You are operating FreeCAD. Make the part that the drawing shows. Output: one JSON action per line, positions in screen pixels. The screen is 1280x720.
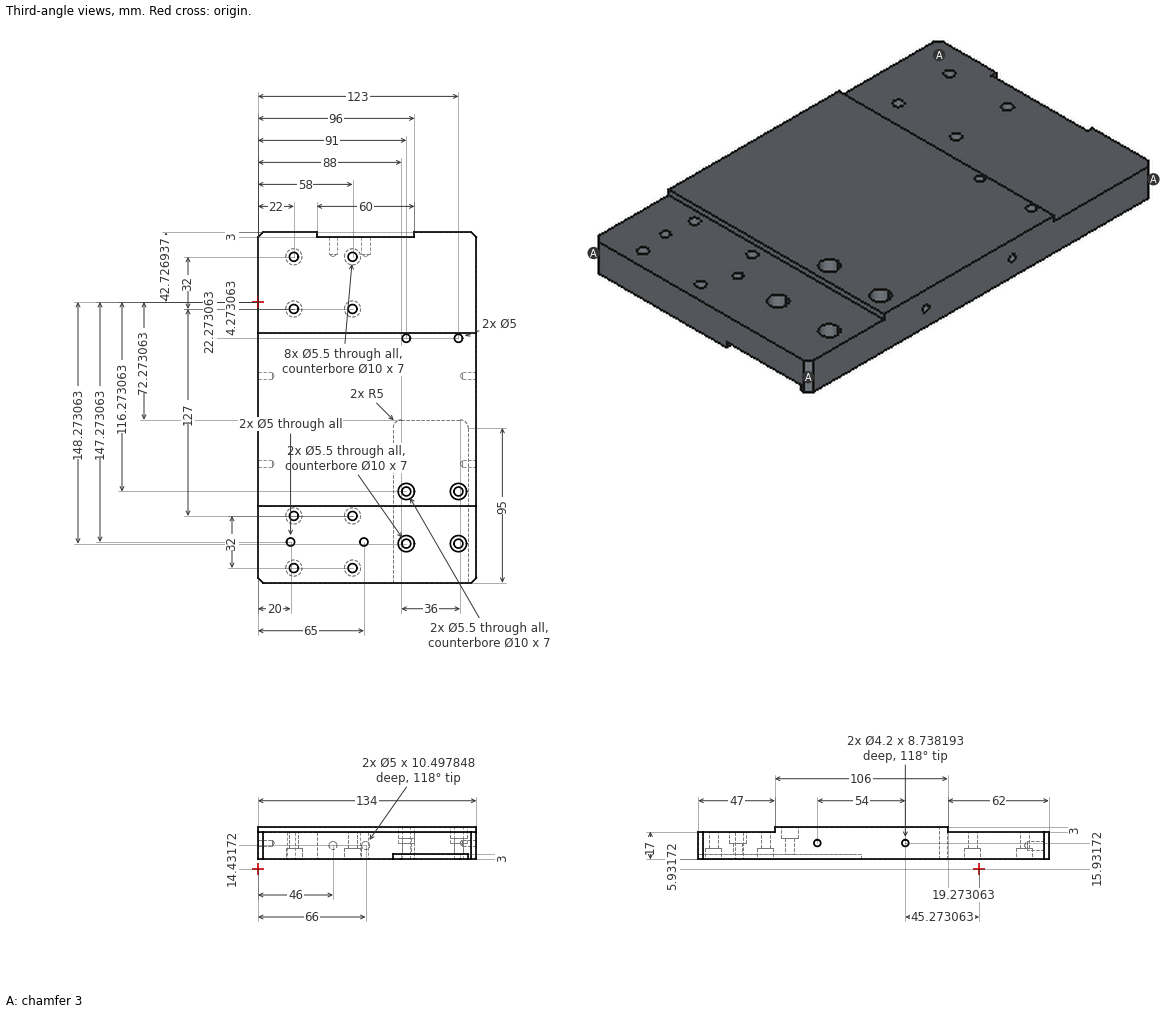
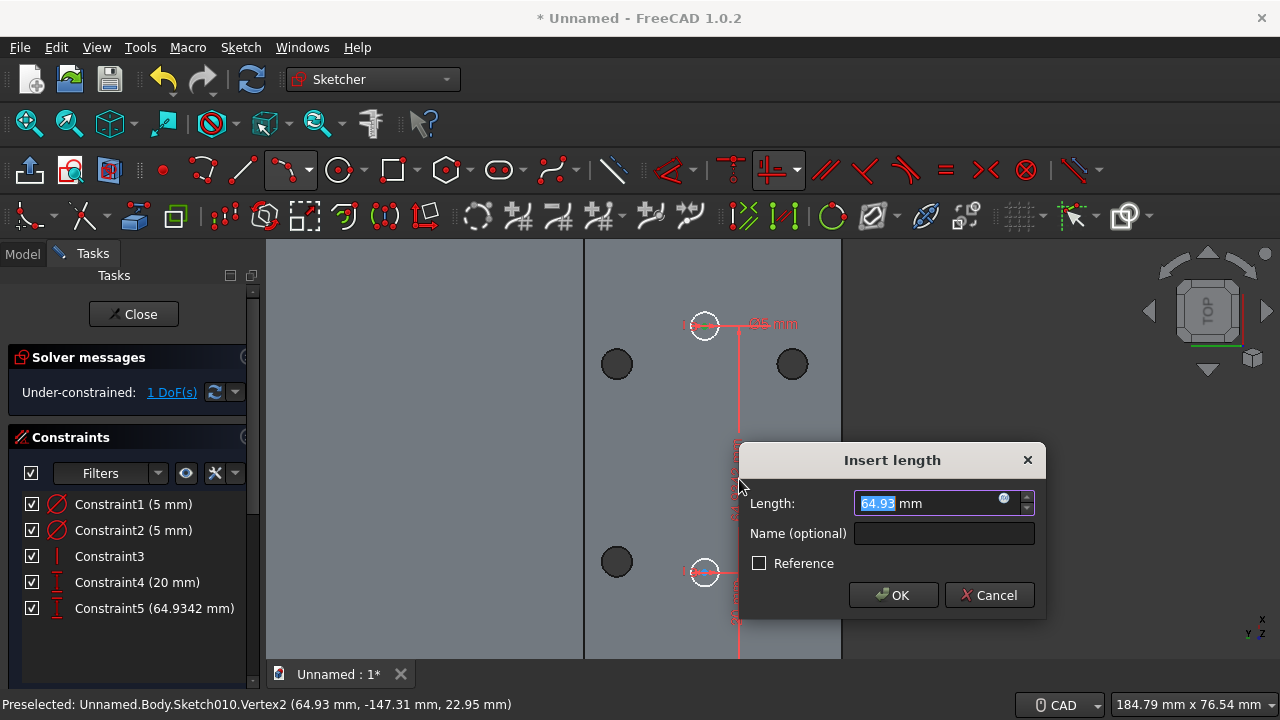
{"action": "type", "text": "65"}
{"action": "key", "text": "Return"}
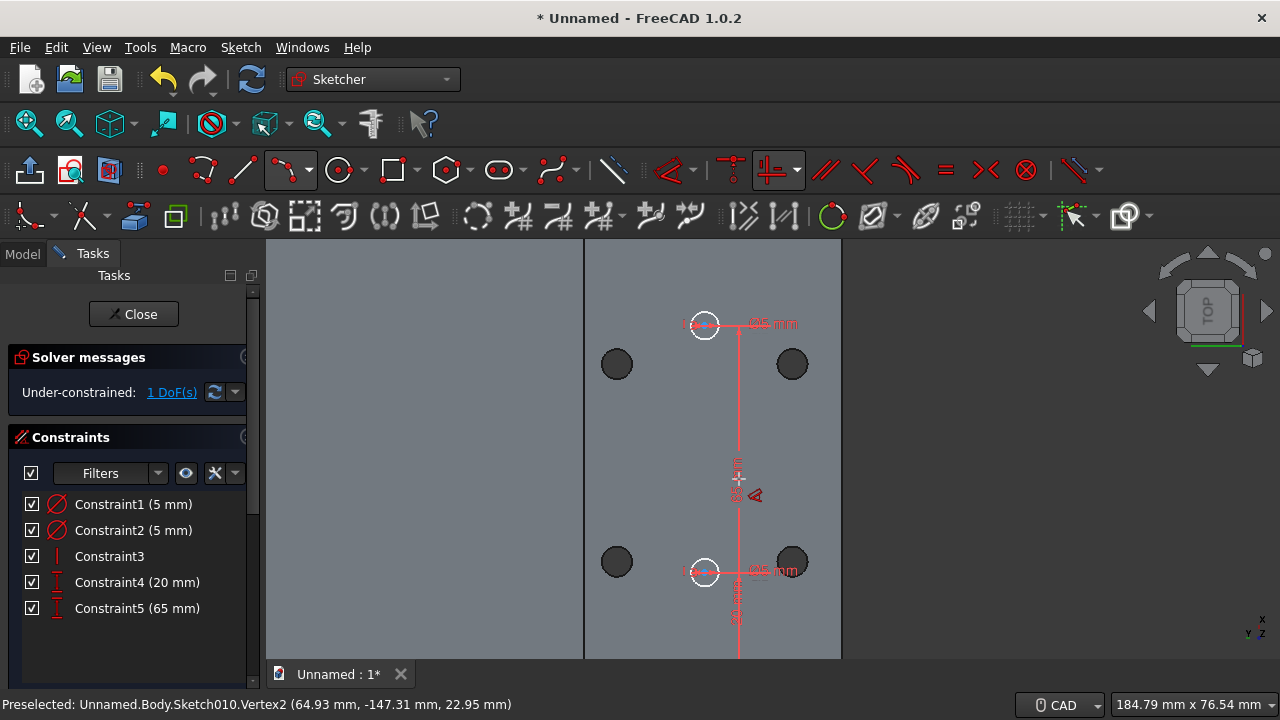
{"action": "left_click", "coordinate": [705, 573]}
{"action": "left_click", "coordinate": [499, 539]}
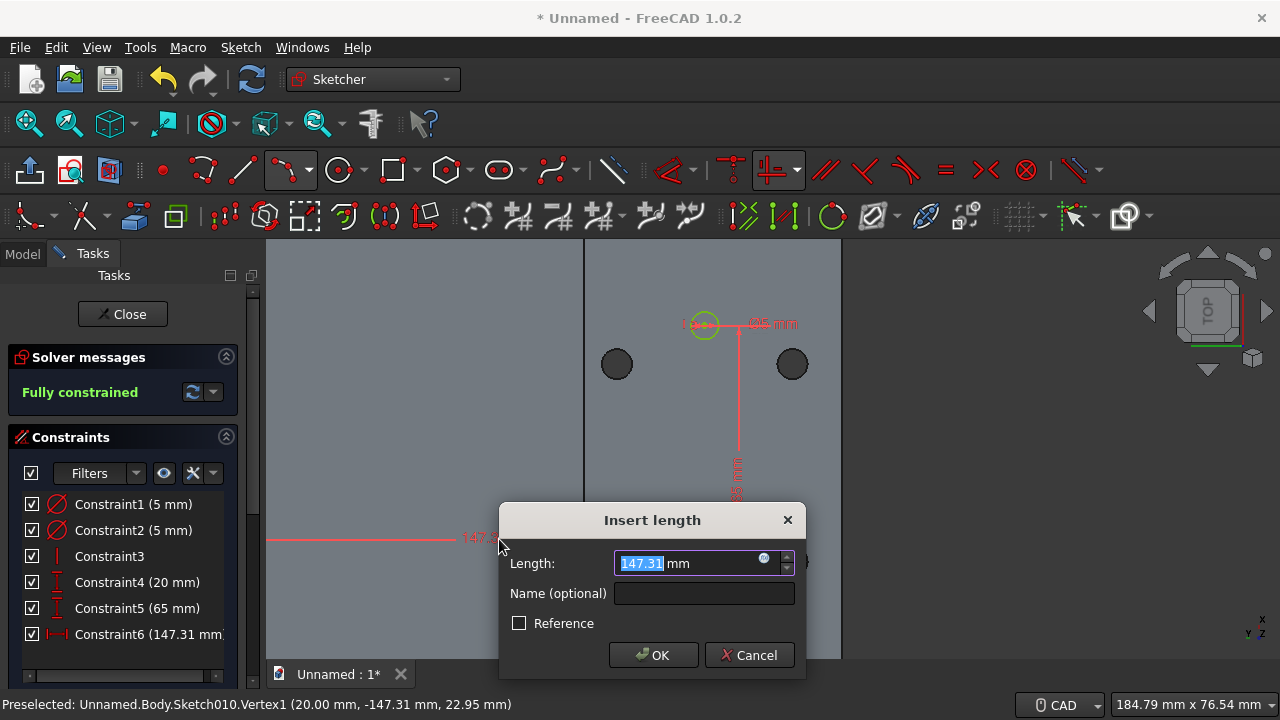
{"action": "type", "text": "147.273063"}
{"action": "key", "text": "Return"}
{"action": "key", "text": "Escape"}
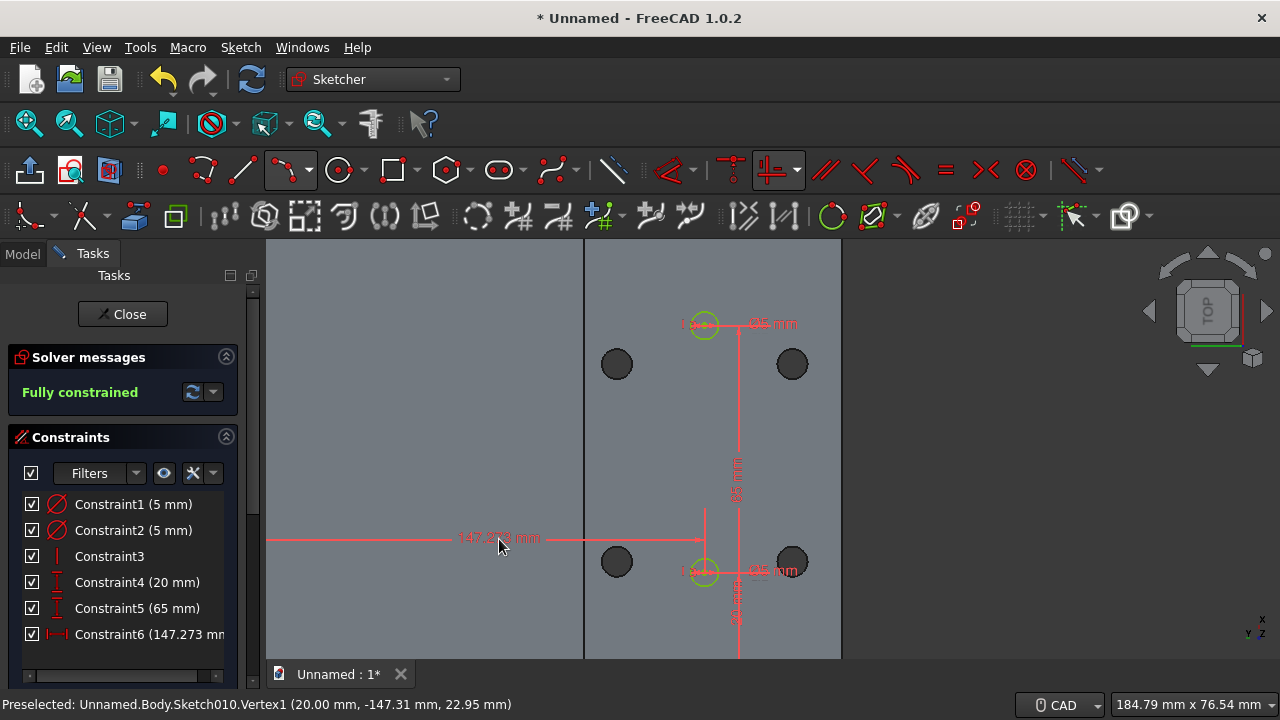
{"action": "left_click", "coordinate": [123, 314]}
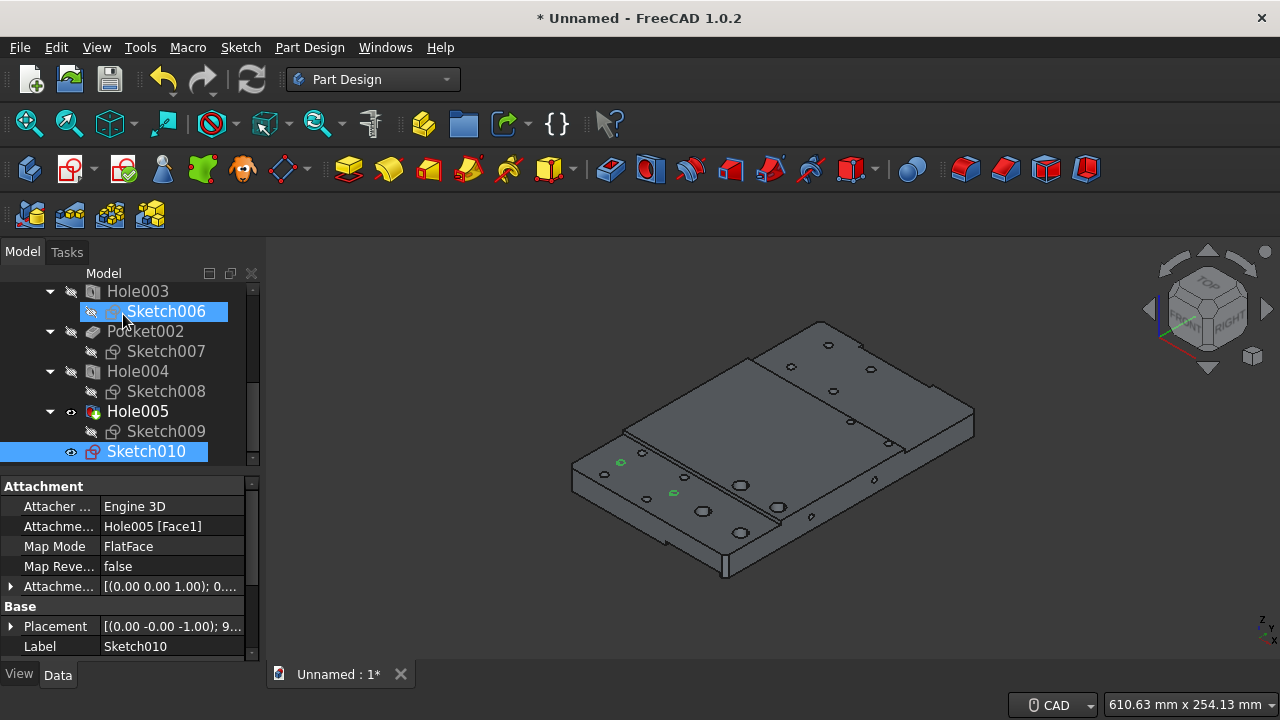
{"action": "left_click", "coordinate": [652, 170]}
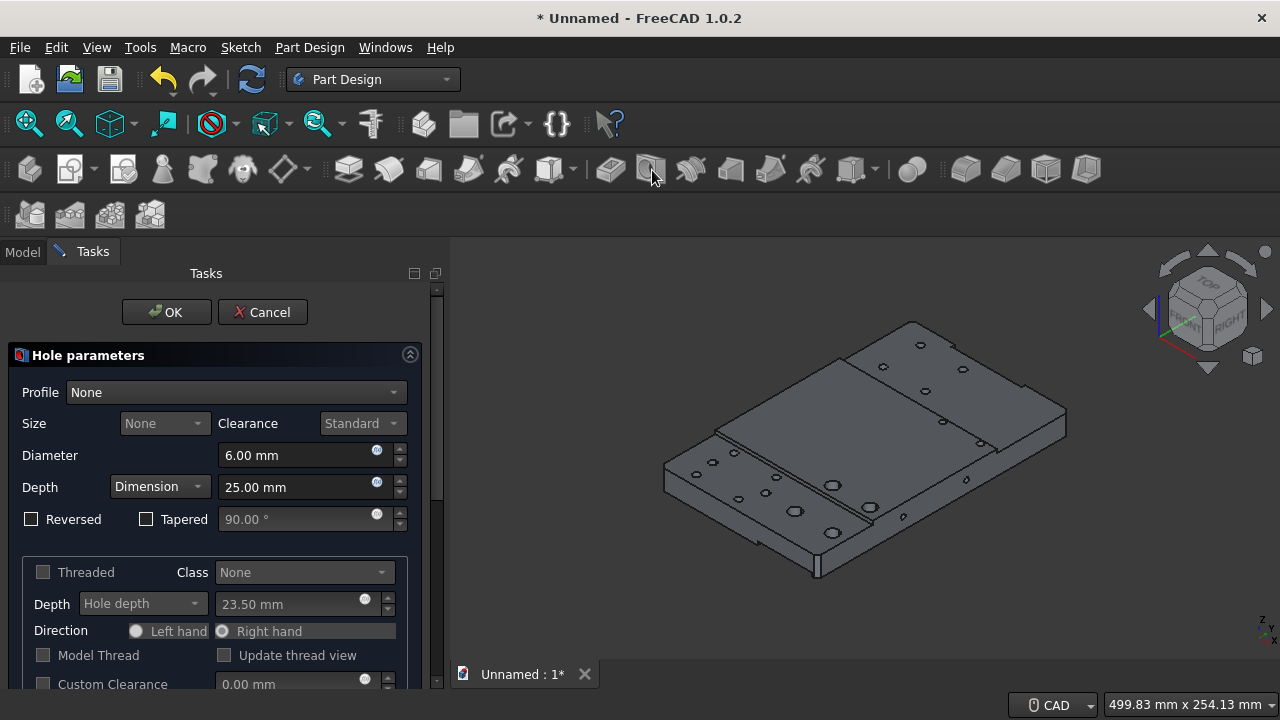
{"action": "triple_click", "coordinate": [305, 455]}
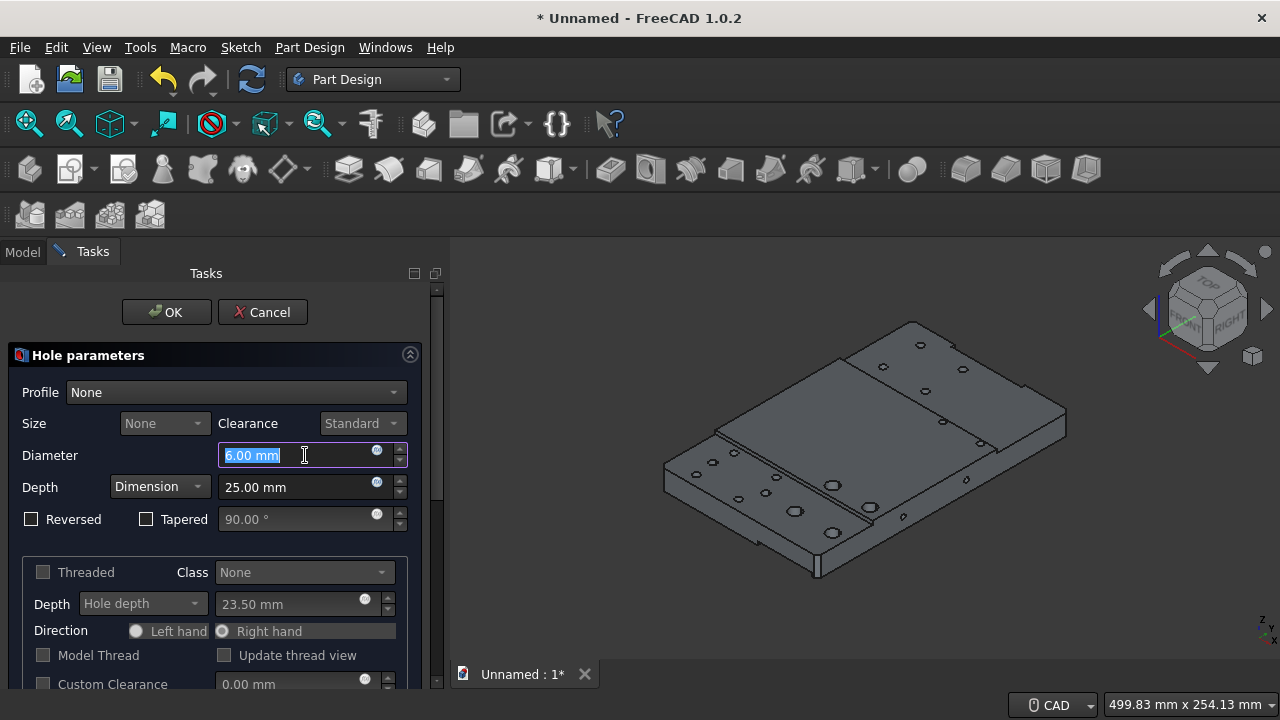
{"action": "type", "text": "5"}
{"action": "key", "text": "Tab"}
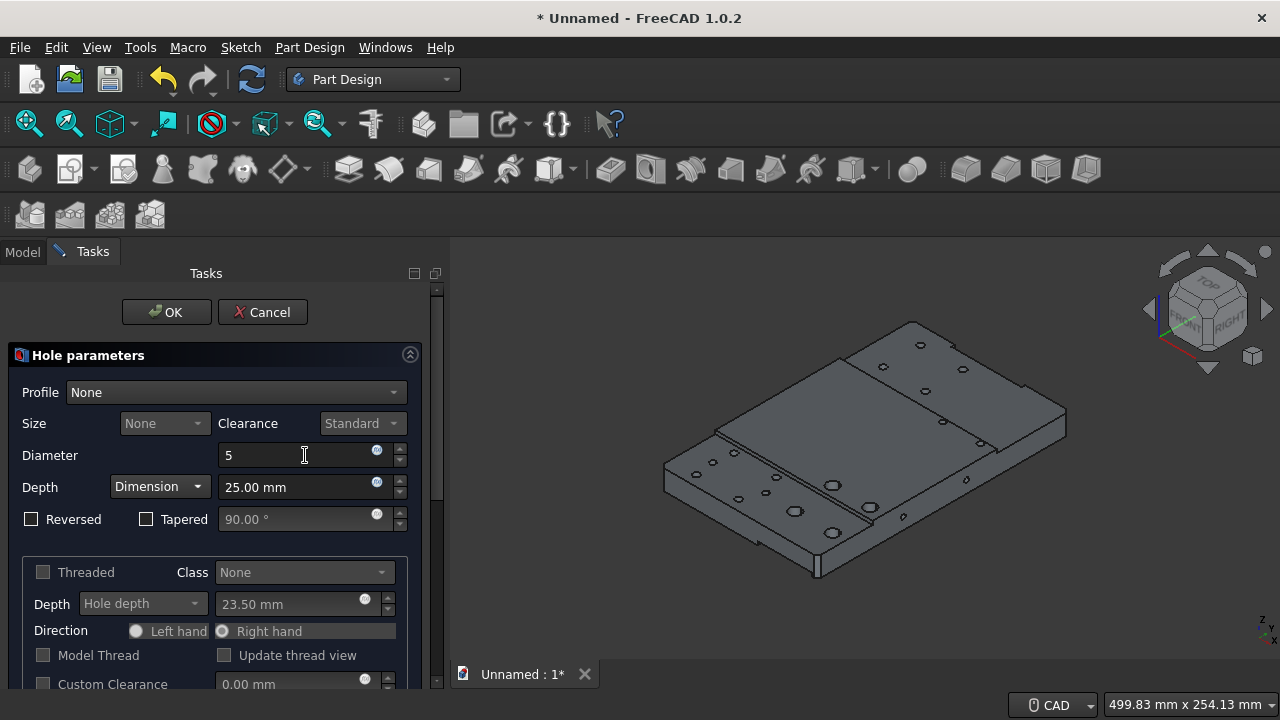
{"action": "left_click", "coordinate": [161, 486]}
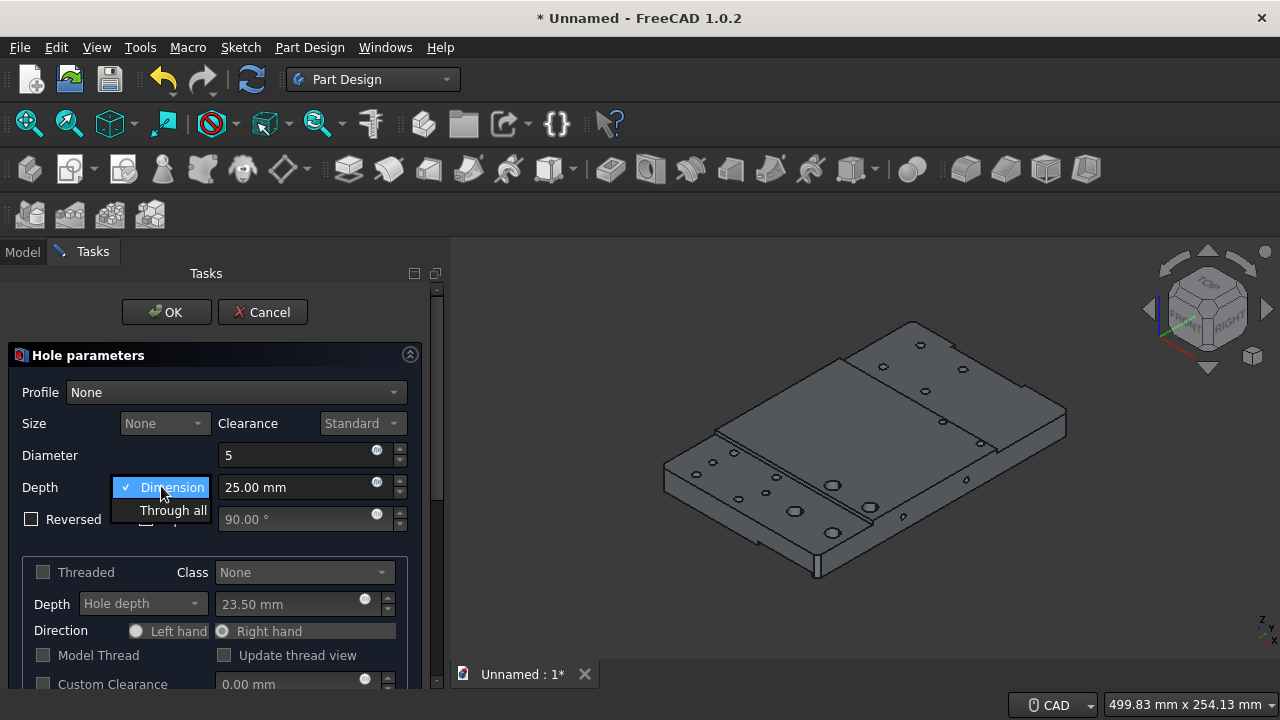
{"action": "left_click", "coordinate": [160, 510]}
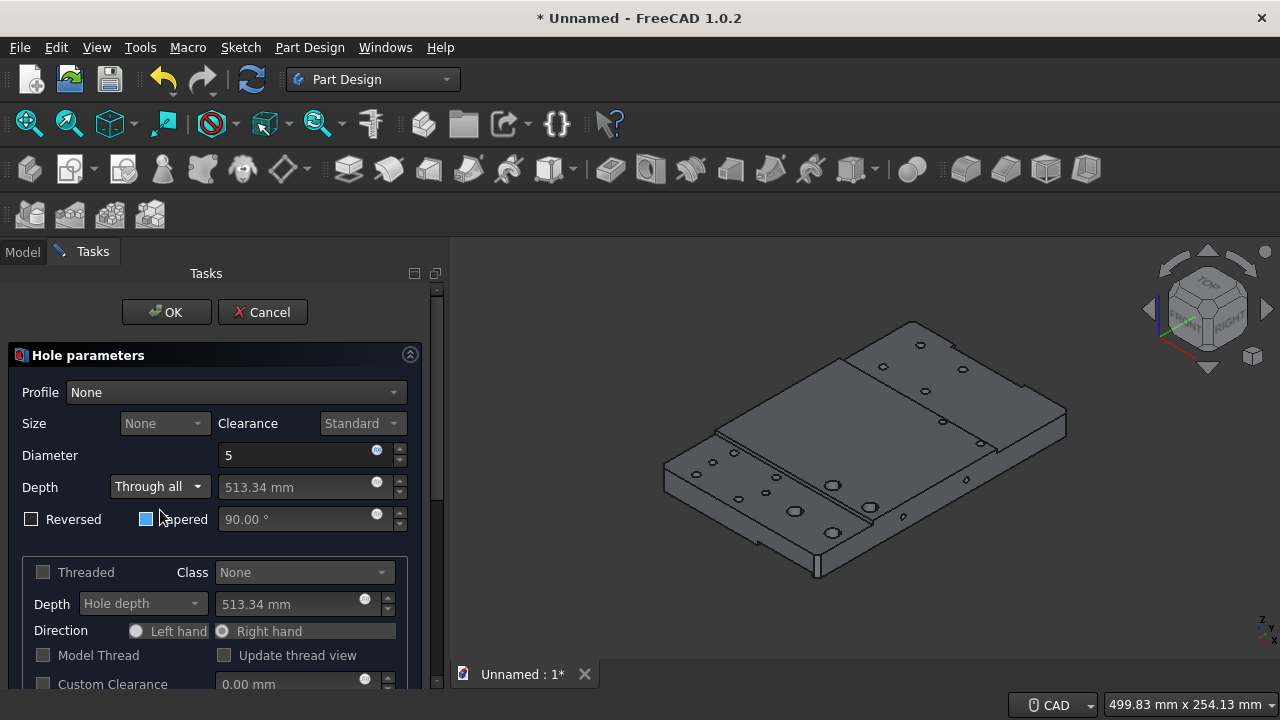
{"action": "left_click", "coordinate": [167, 312]}